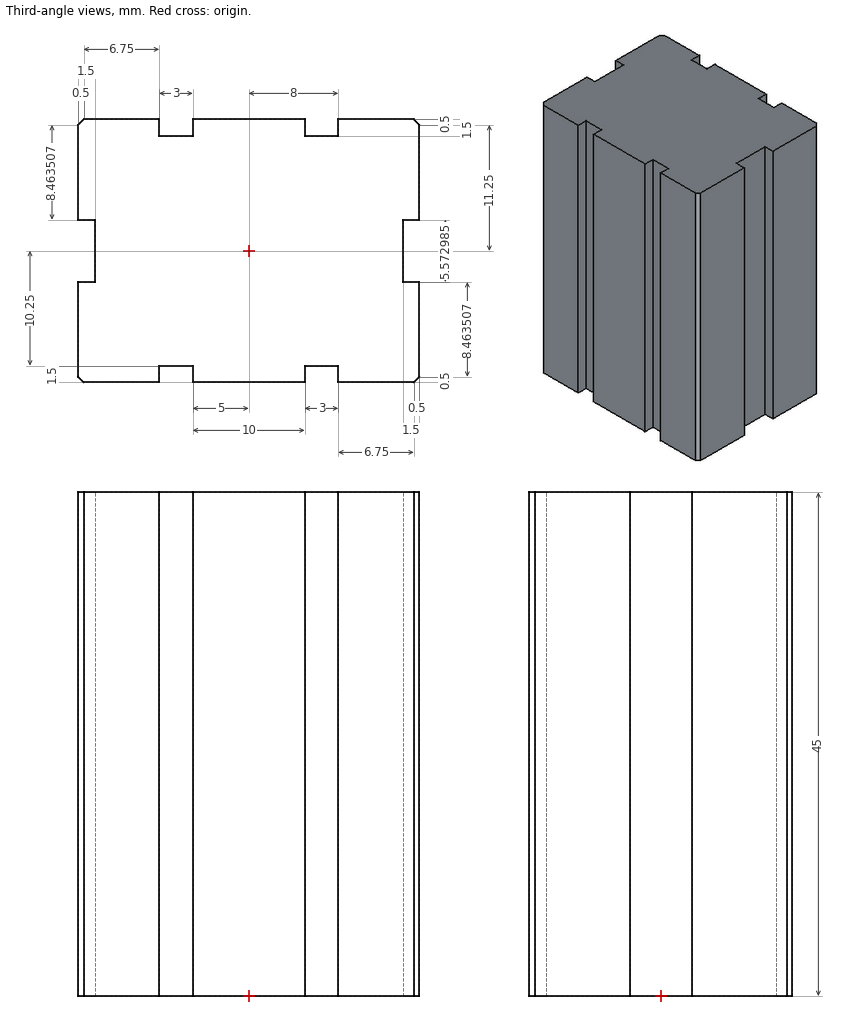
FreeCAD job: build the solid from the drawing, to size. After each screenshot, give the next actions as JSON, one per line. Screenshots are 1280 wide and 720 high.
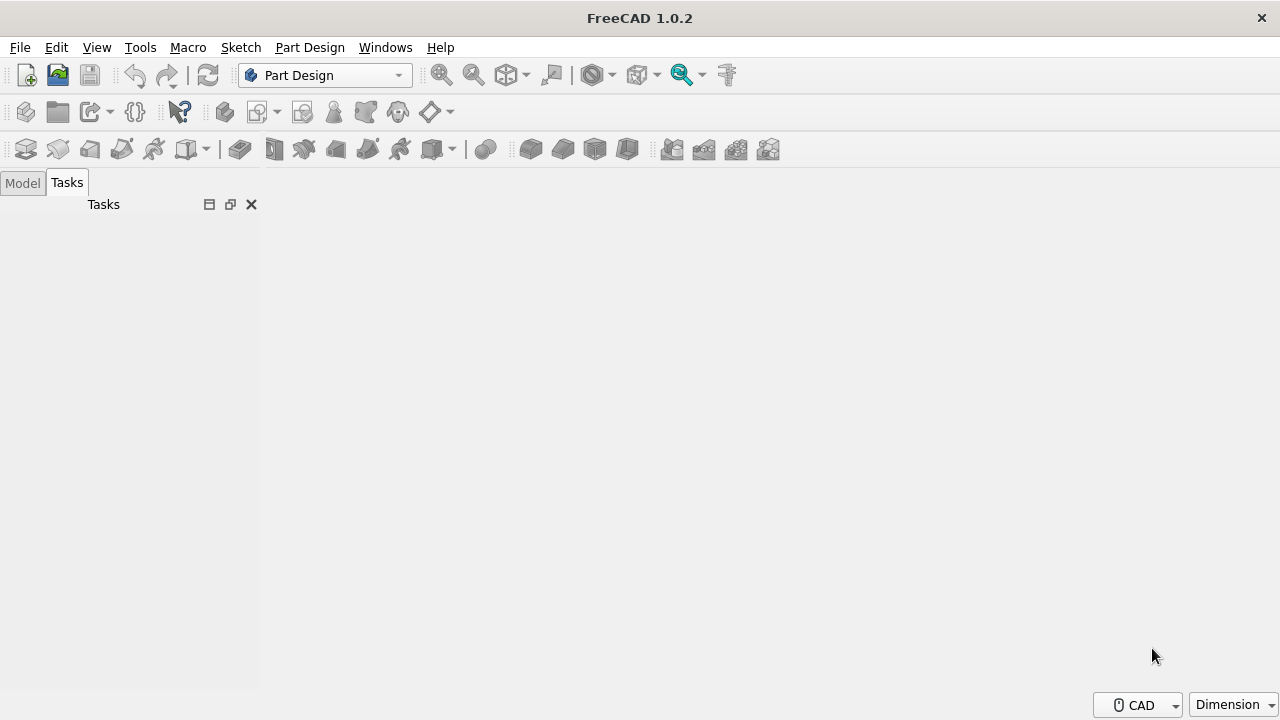
{"action": "key", "text": "ctrl+n"}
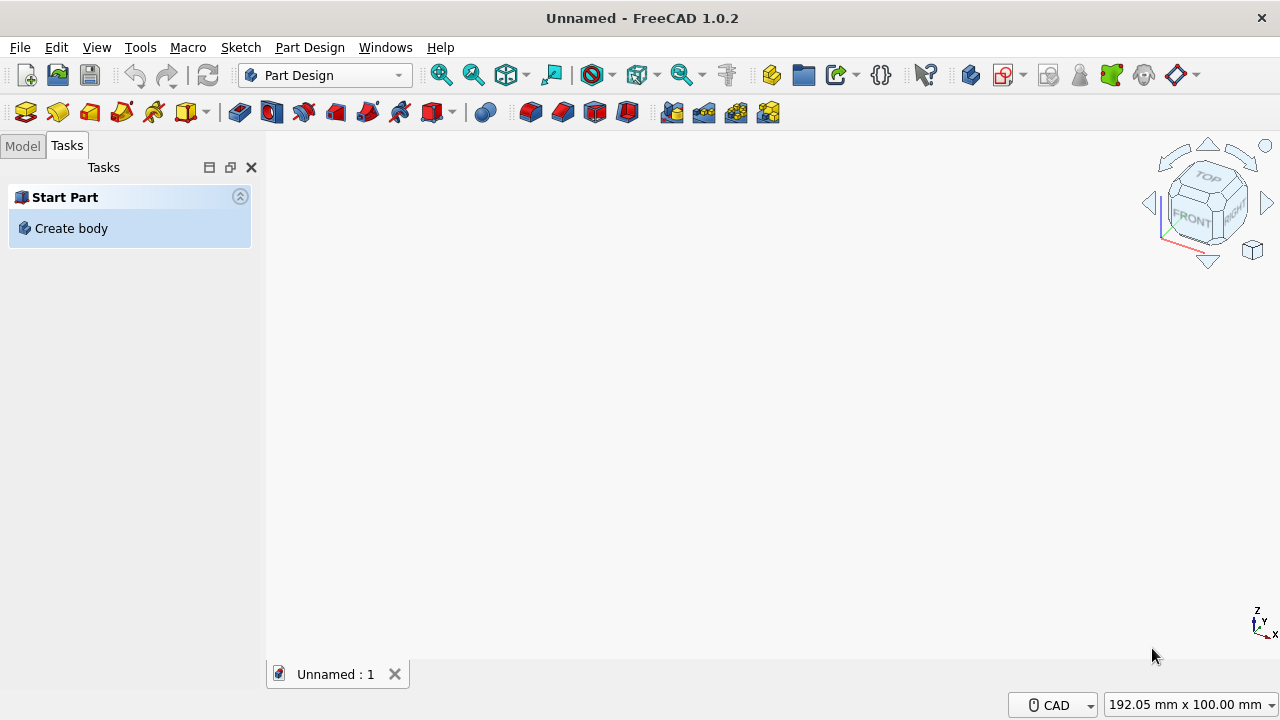
{"action": "left_click", "coordinate": [1004, 76]}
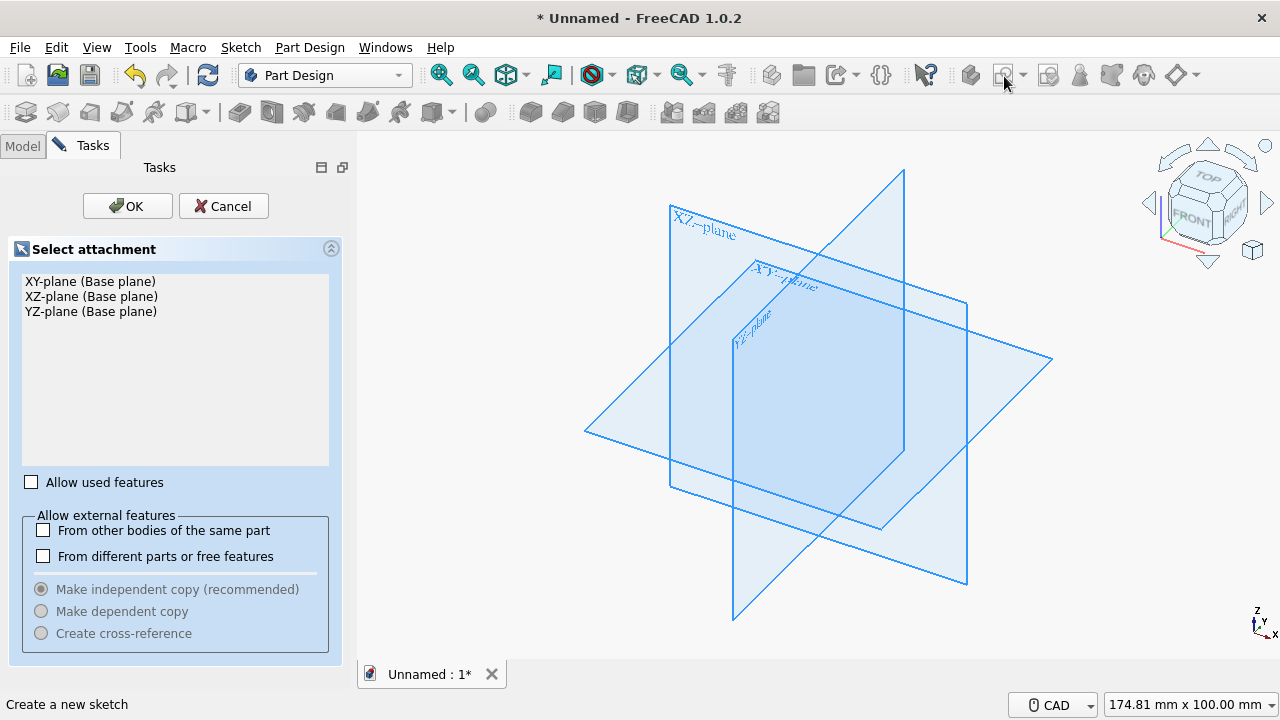
{"action": "left_click", "coordinate": [82, 282]}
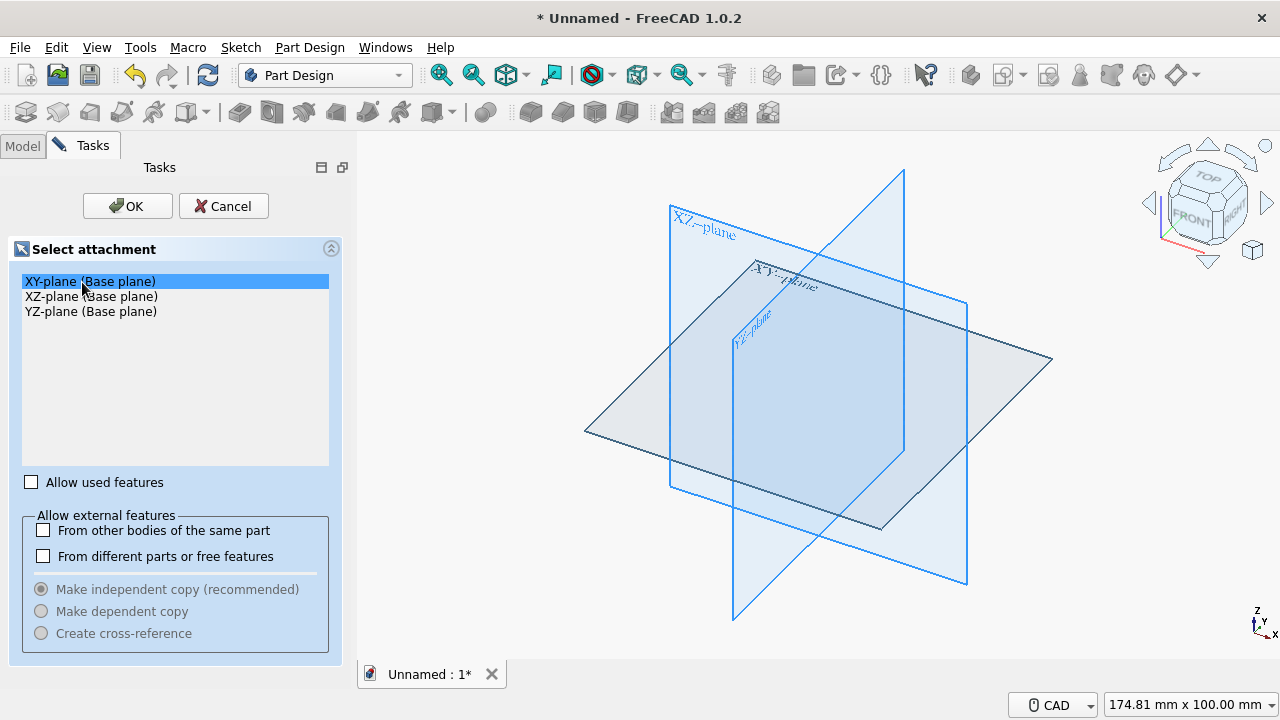
{"action": "left_click", "coordinate": [128, 206]}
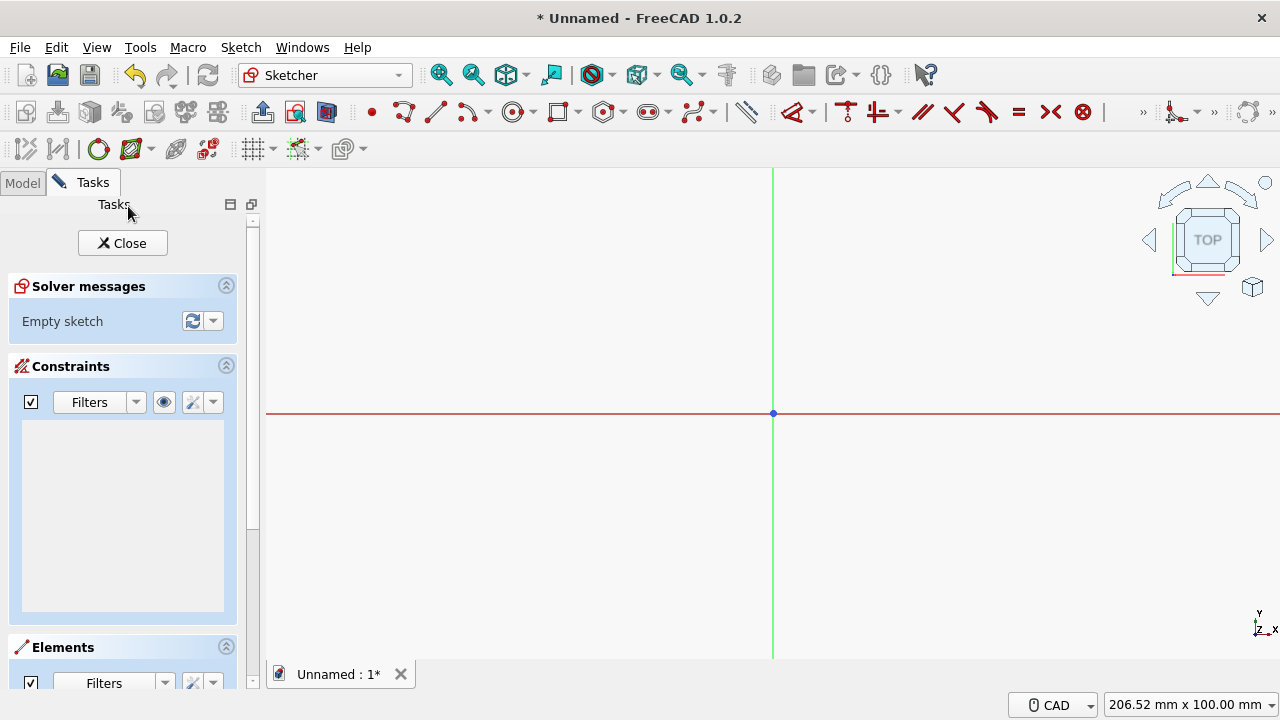
{"action": "scroll", "coordinate": [813, 414], "scroll_direction": "up", "scroll_amount": 5}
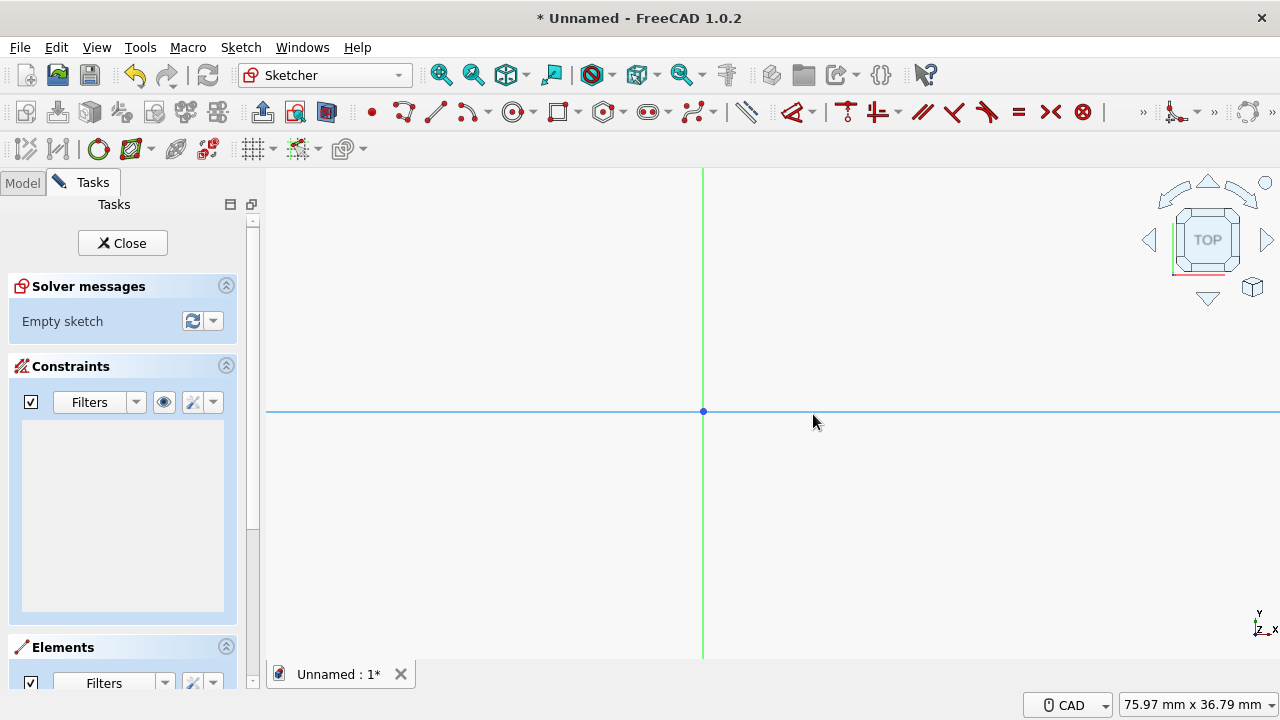
{"action": "key", "text": "g m"}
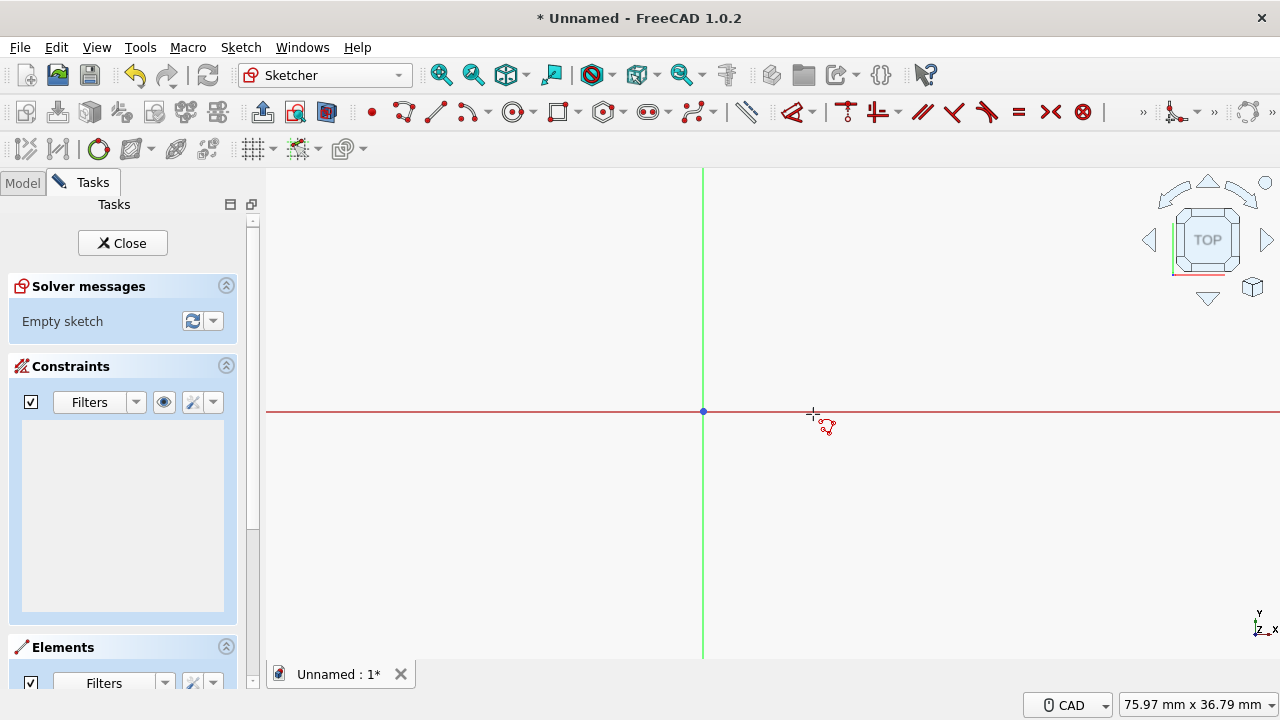
{"action": "left_click", "coordinate": [637, 549]}
{"action": "left_click", "coordinate": [637, 569]}
{"action": "left_click", "coordinate": [770, 569]}
{"action": "left_click", "coordinate": [770, 549]}
{"action": "left_click", "coordinate": [810, 549]}
{"action": "left_click", "coordinate": [810, 569]}
{"action": "left_click", "coordinate": [900, 569]}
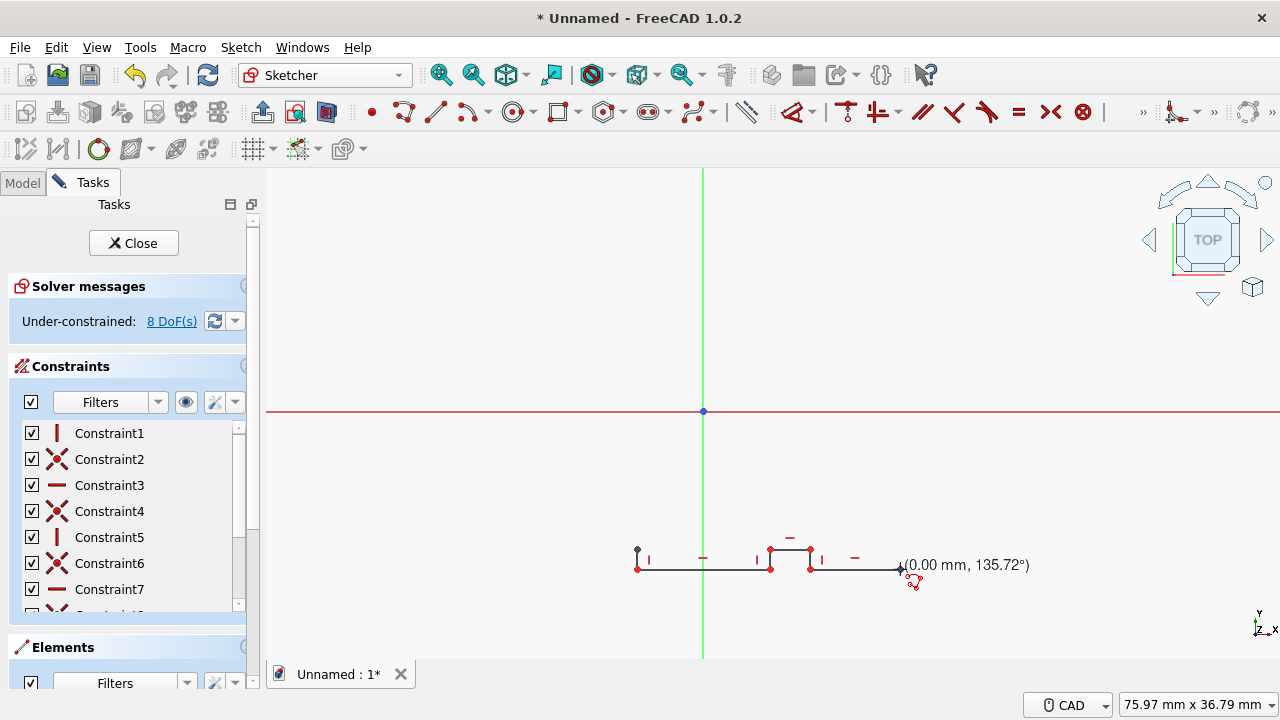
{"action": "scroll", "coordinate": [907, 562], "scroll_direction": "up", "scroll_amount": 3}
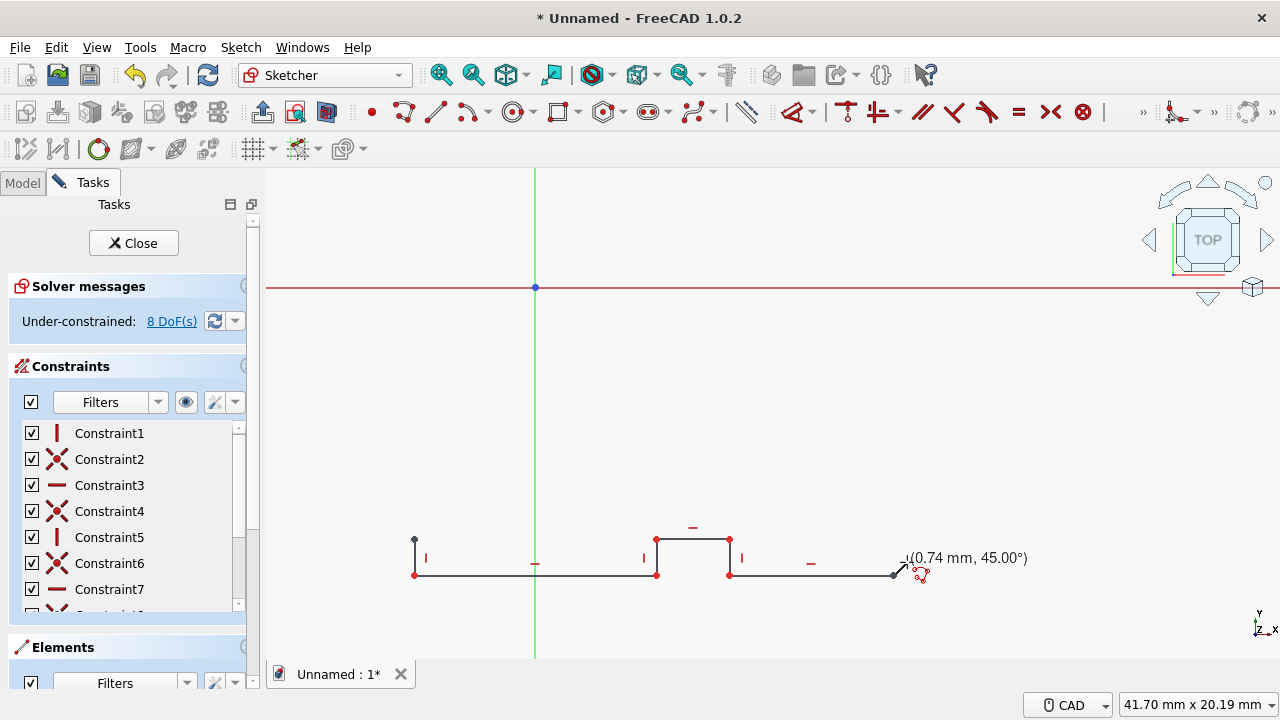
{"action": "left_click", "coordinate": [906, 561]}
{"action": "left_click", "coordinate": [906, 355]}
{"action": "left_click", "coordinate": [870, 355]}
{"action": "left_click", "coordinate": [870, 220]}
{"action": "left_click", "coordinate": [906, 220]}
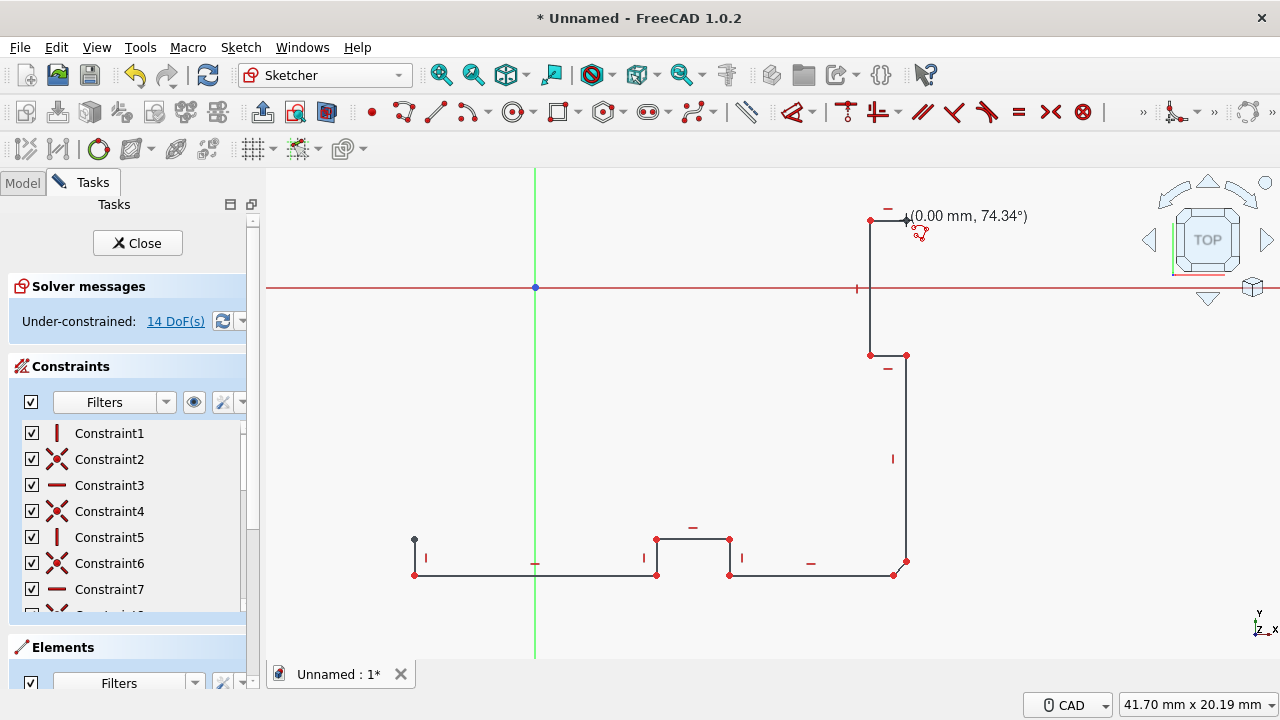
{"action": "scroll", "coordinate": [910, 567], "scroll_direction": "down", "scroll_amount": 3}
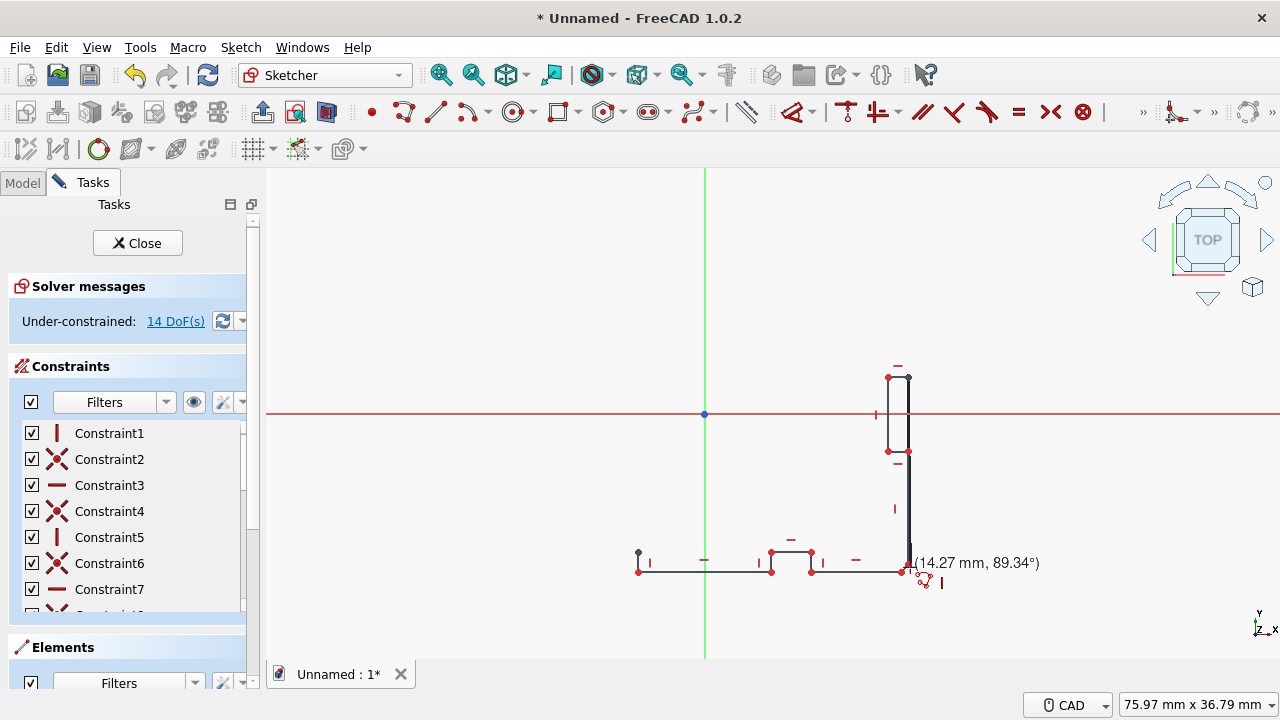
{"action": "left_click", "coordinate": [908, 264]}